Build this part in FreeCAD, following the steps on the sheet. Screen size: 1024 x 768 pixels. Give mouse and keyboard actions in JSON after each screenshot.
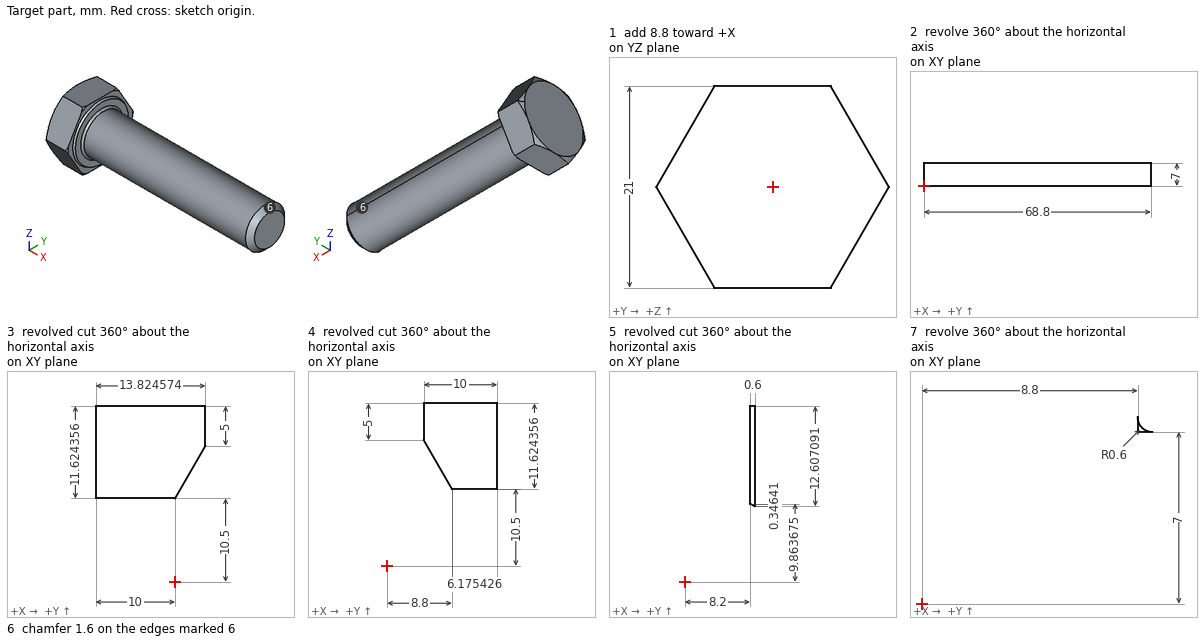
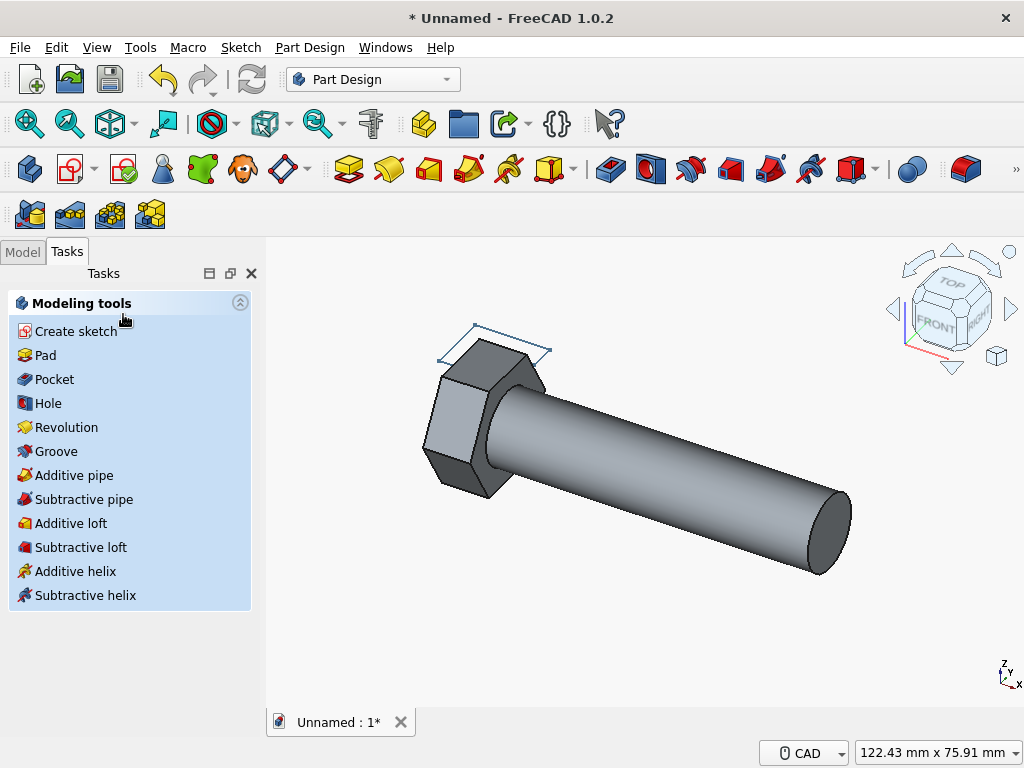
{"action": "left_click", "coordinate": [692, 170]}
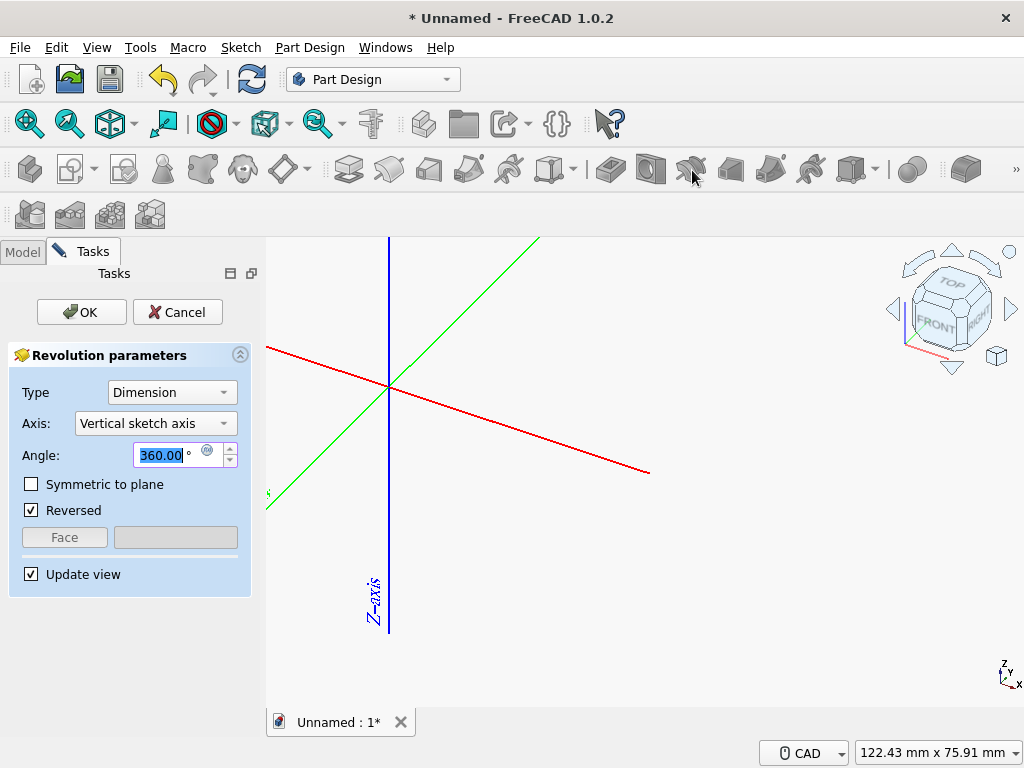
{"action": "left_click", "coordinate": [156, 424]}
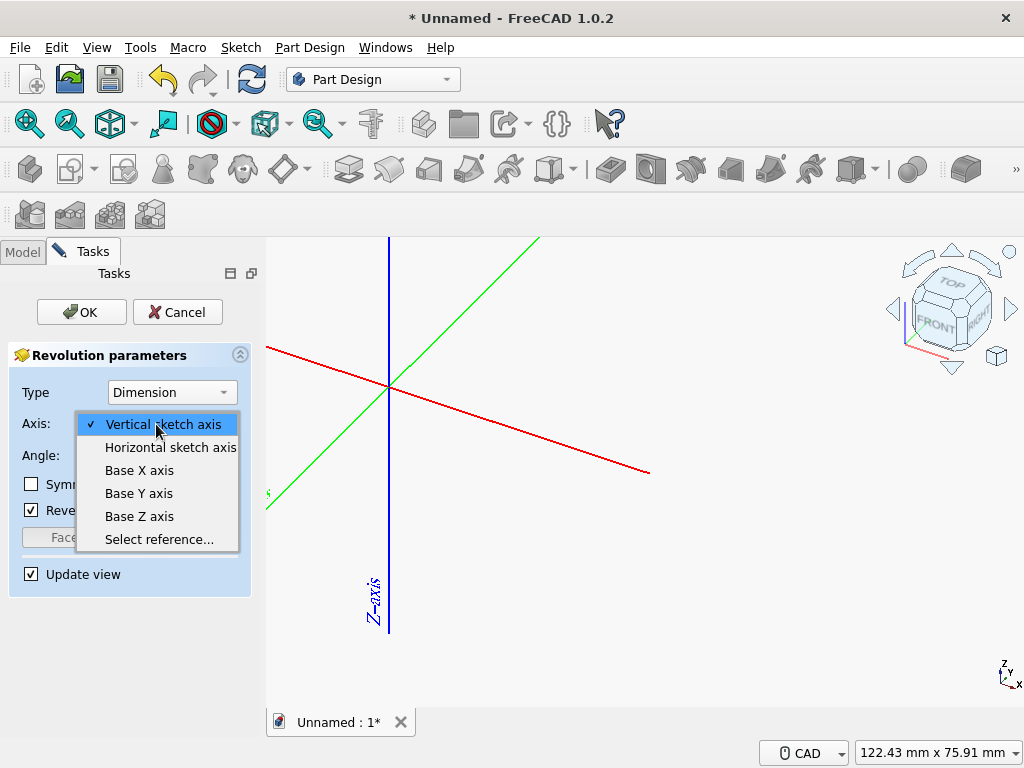
{"action": "left_click", "coordinate": [156, 448]}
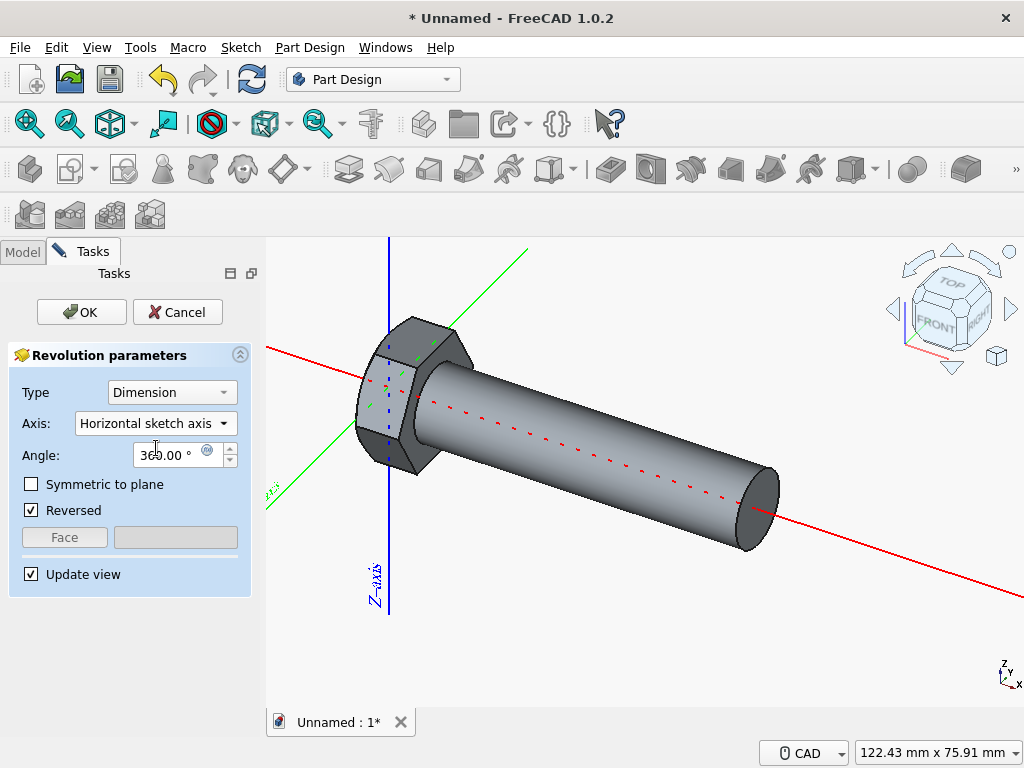
{"action": "left_click", "coordinate": [82, 312]}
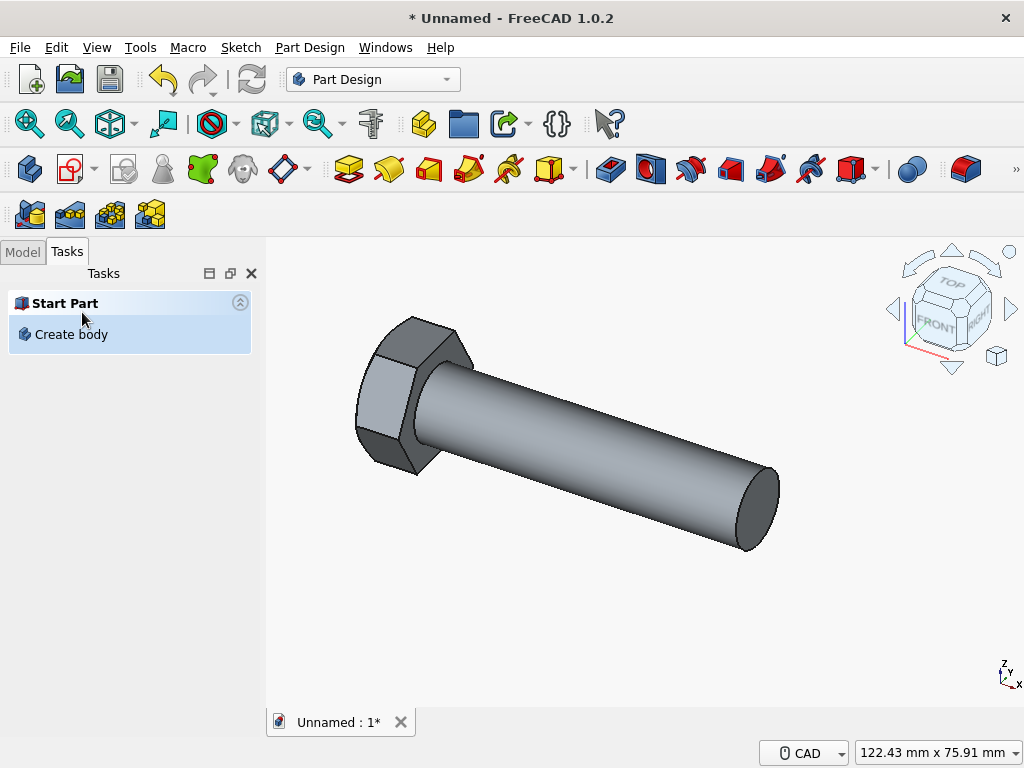
{"action": "left_click", "coordinate": [70, 170]}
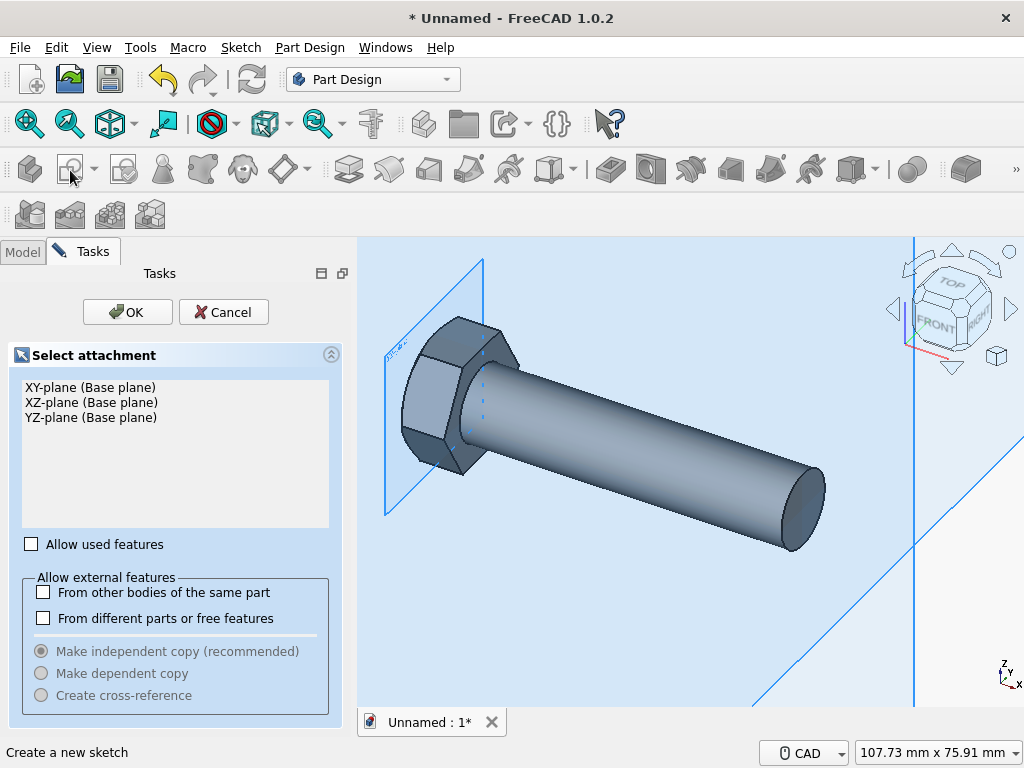
{"action": "left_click", "coordinate": [82, 388]}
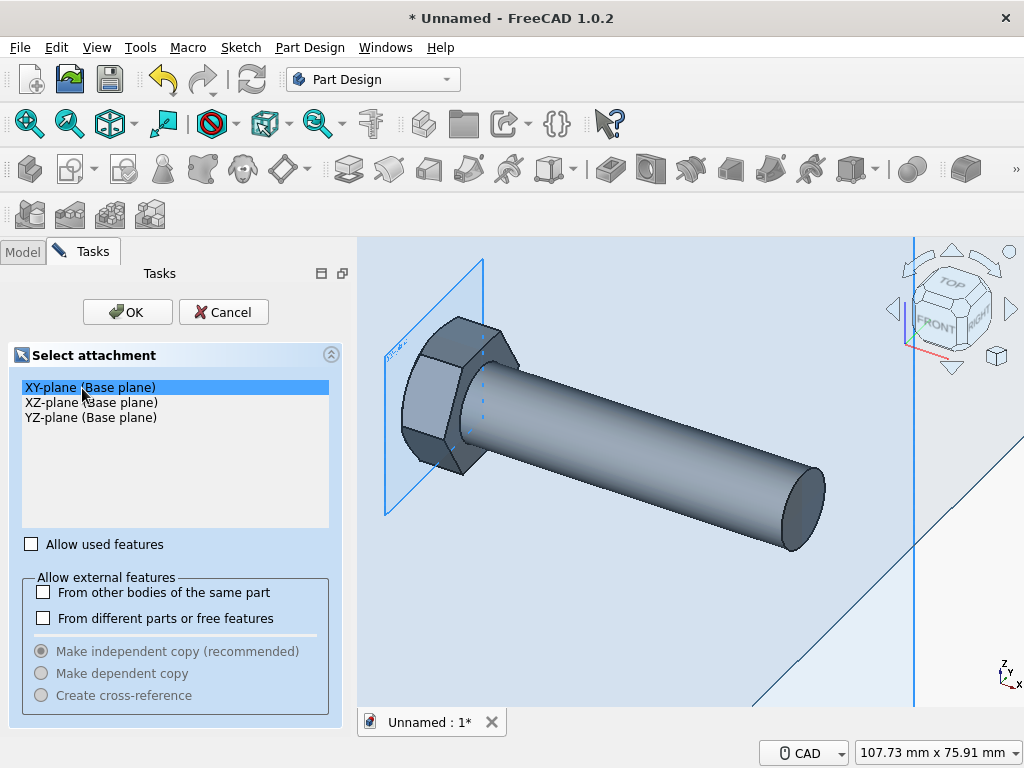
{"action": "left_click", "coordinate": [128, 312]}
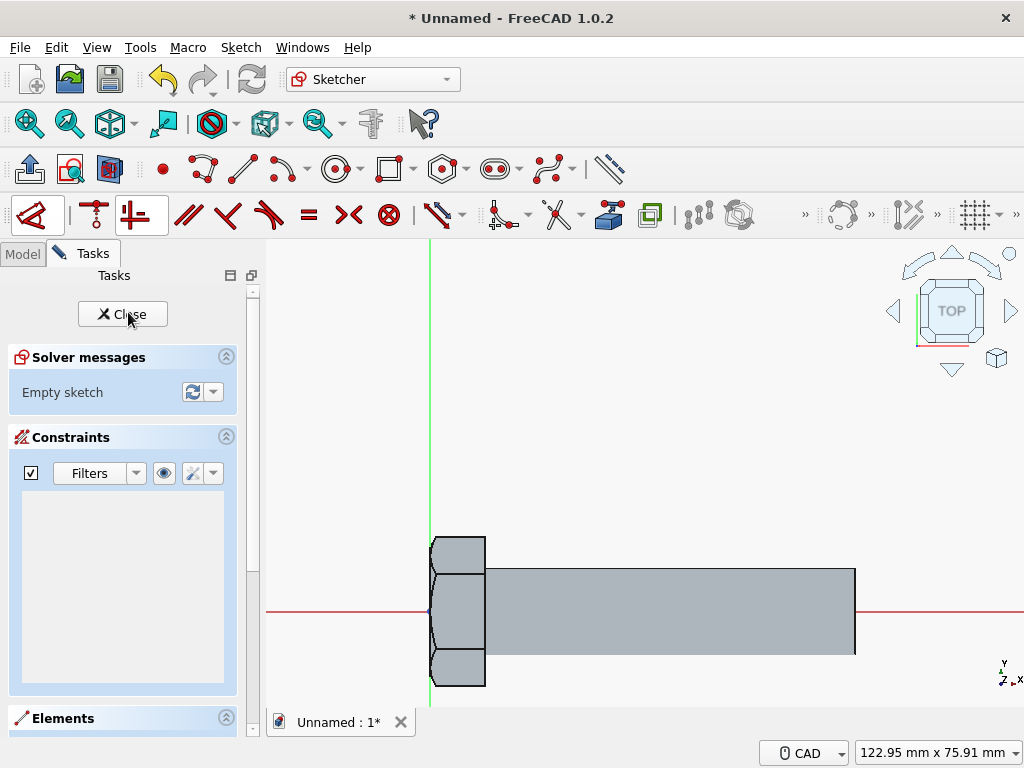
{"action": "left_click", "coordinate": [110, 170]}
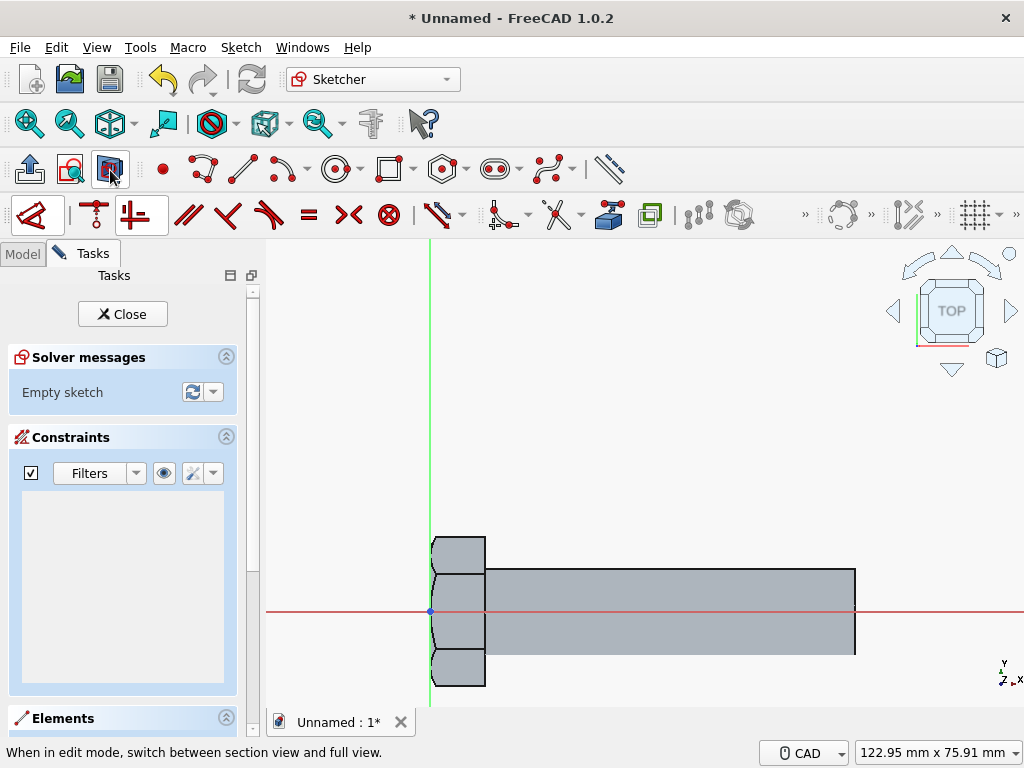
{"action": "scroll", "coordinate": [395, 601], "scroll_direction": "up", "scroll_amount": 4}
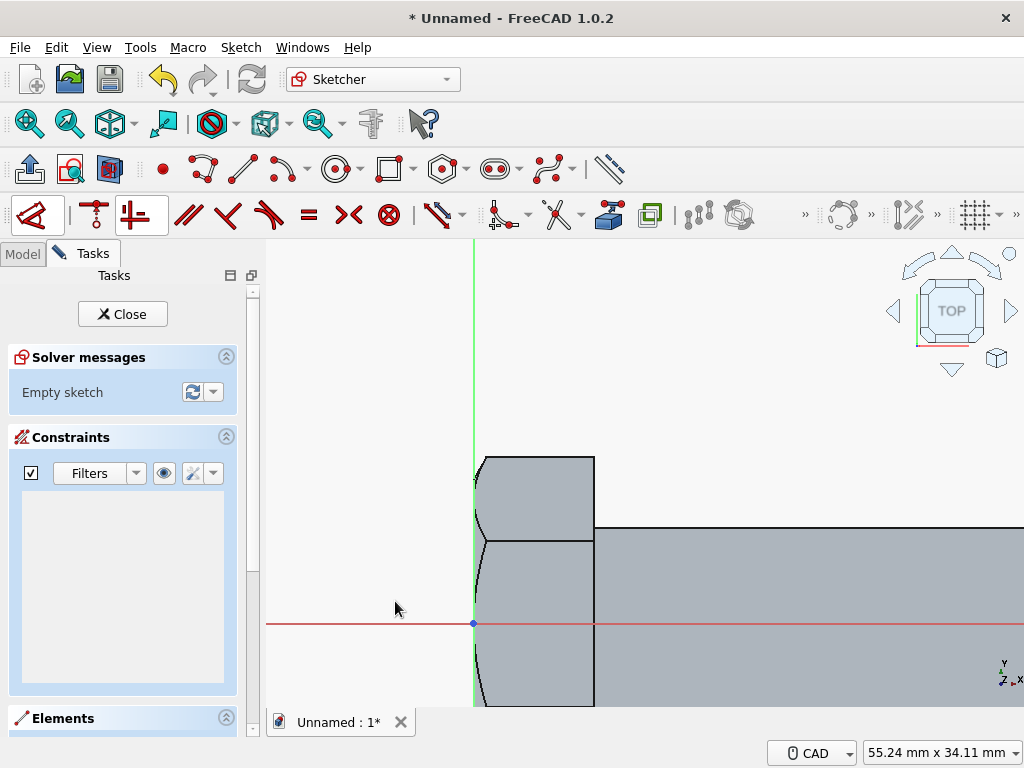
{"action": "left_click", "coordinate": [204, 170]}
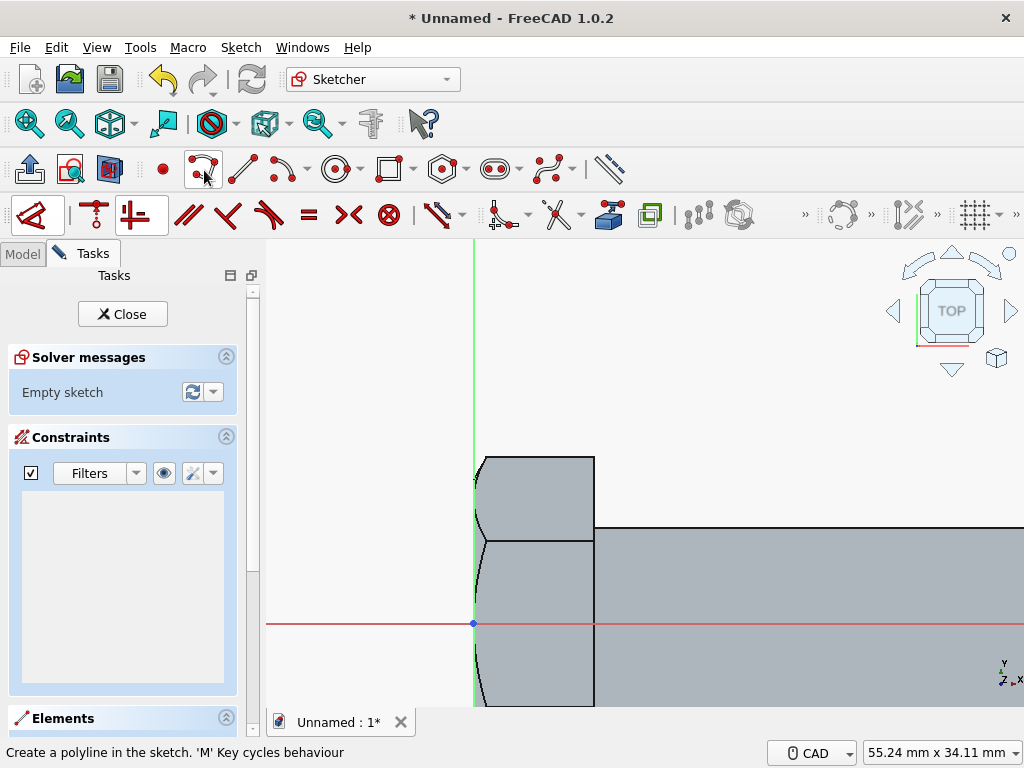
{"action": "left_click", "coordinate": [594, 480]}
{"action": "left_click", "coordinate": [679, 480]}
{"action": "left_click", "coordinate": [679, 320]}
{"action": "left_click", "coordinate": [542, 320]}
{"action": "left_click", "coordinate": [542, 389]}
{"action": "left_click", "coordinate": [594, 481]}
{"action": "key", "text": "Escape"}
{"action": "key", "text": "Escape"}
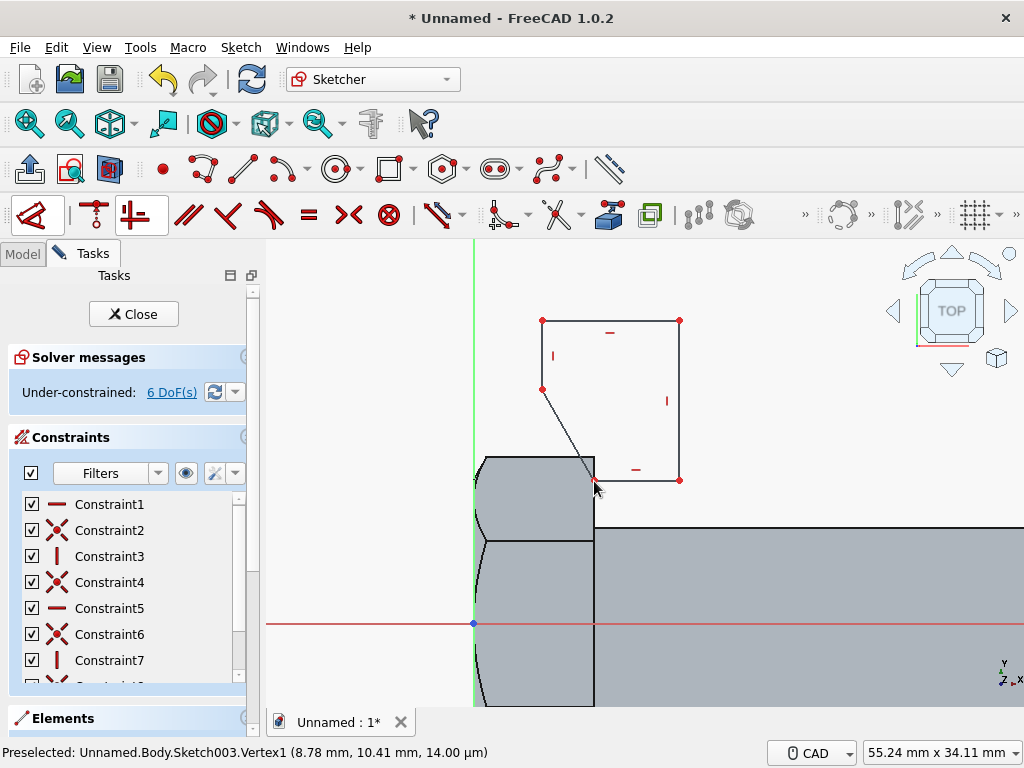
{"action": "left_click", "coordinate": [542, 342]}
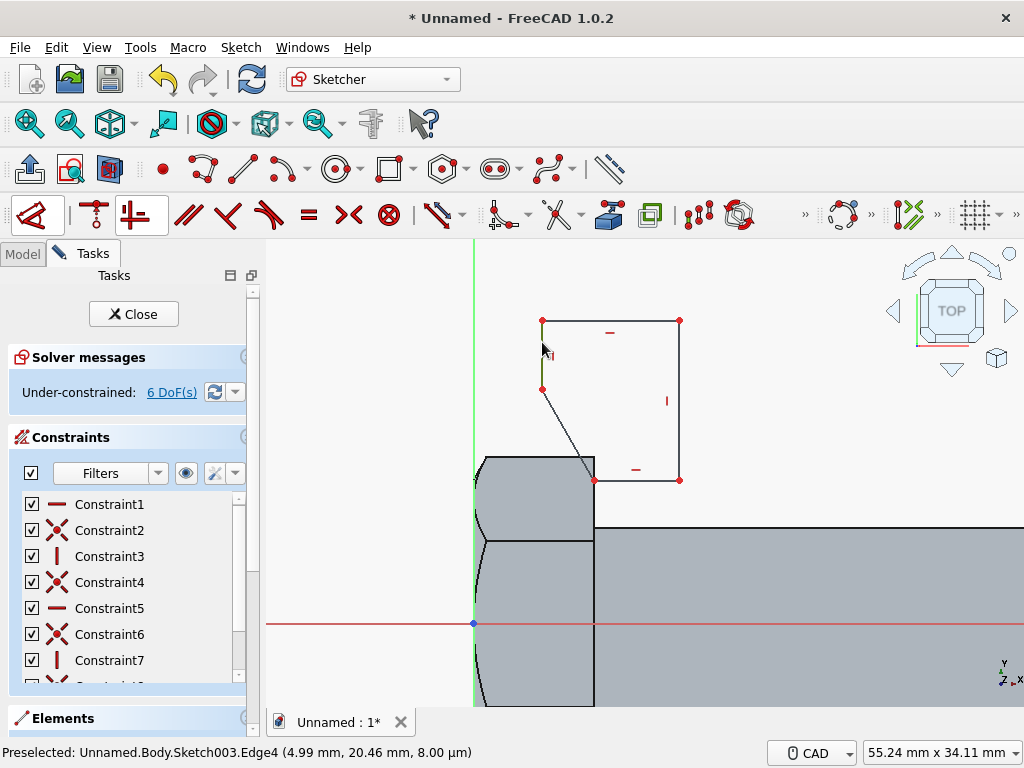
{"action": "left_click", "coordinate": [58, 216]}